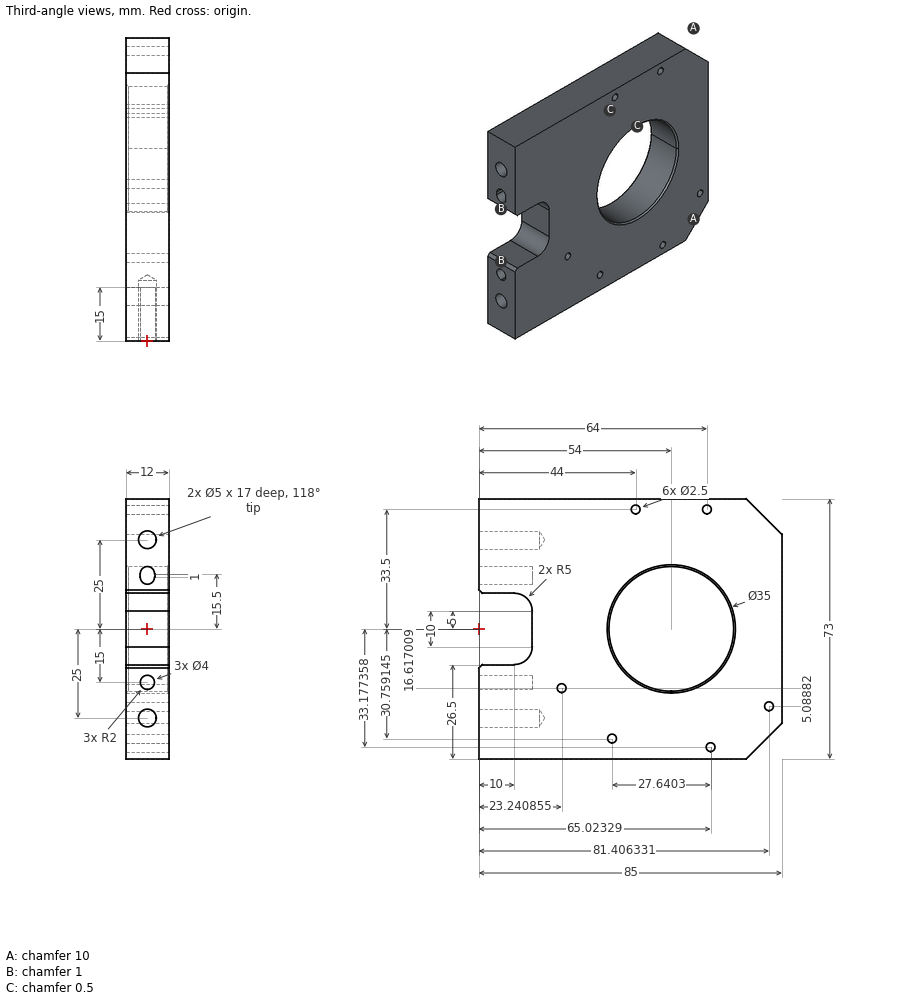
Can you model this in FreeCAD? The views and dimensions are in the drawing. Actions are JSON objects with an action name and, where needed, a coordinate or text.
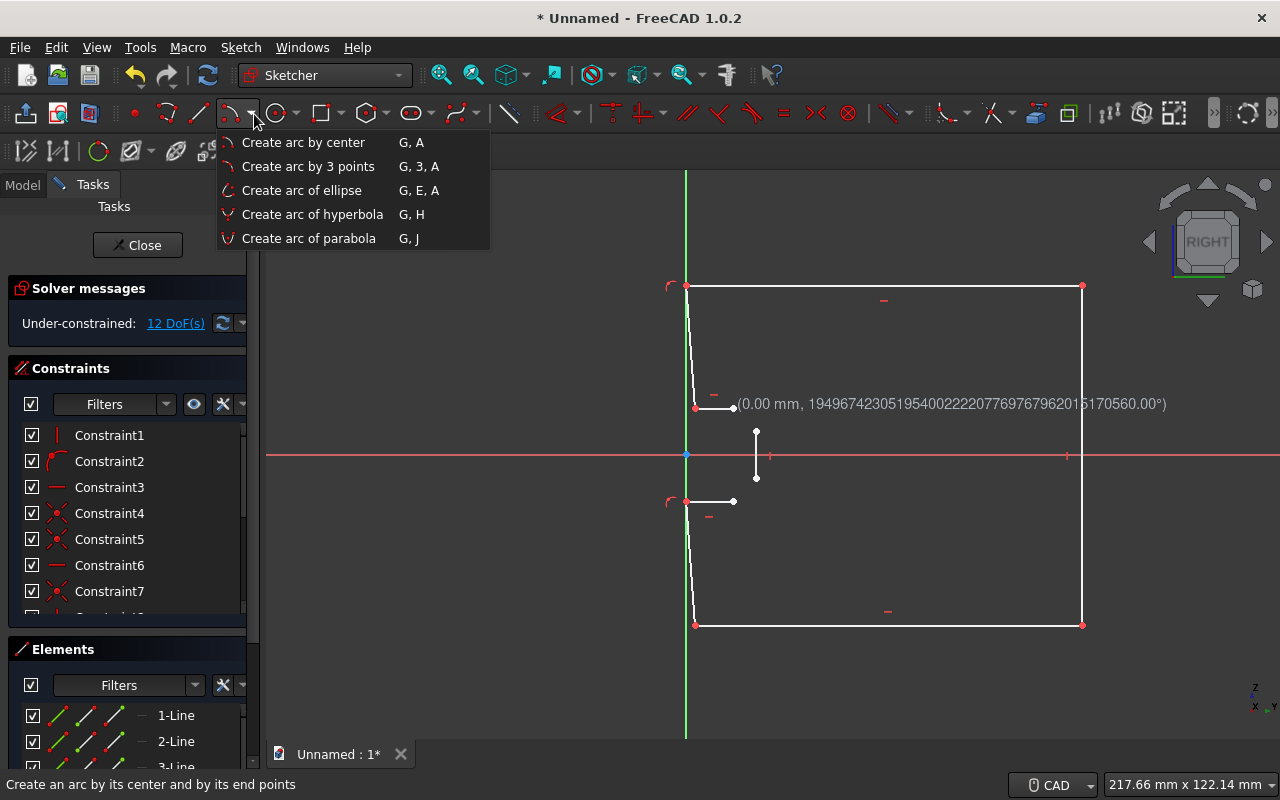
{"action": "left_click", "coordinate": [354, 166]}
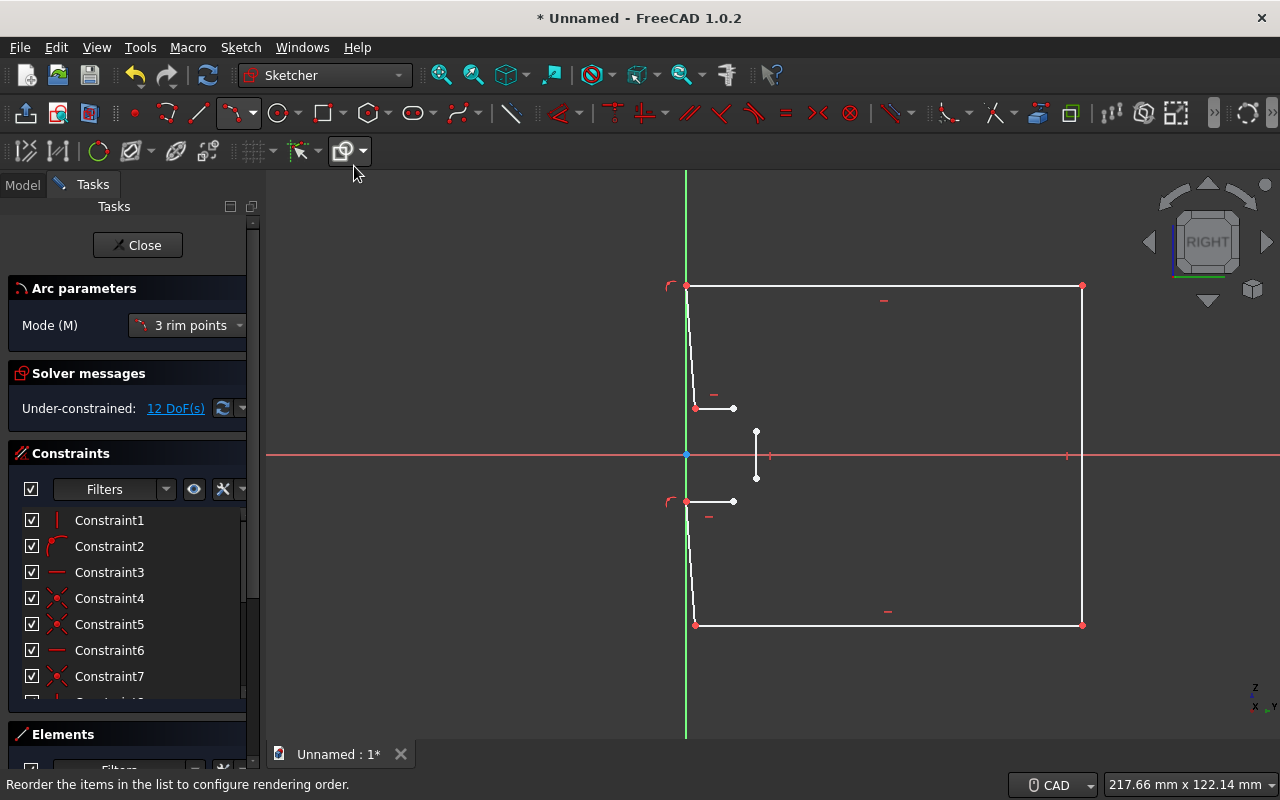
{"action": "left_click", "coordinate": [756, 479]}
{"action": "left_click", "coordinate": [733, 502]}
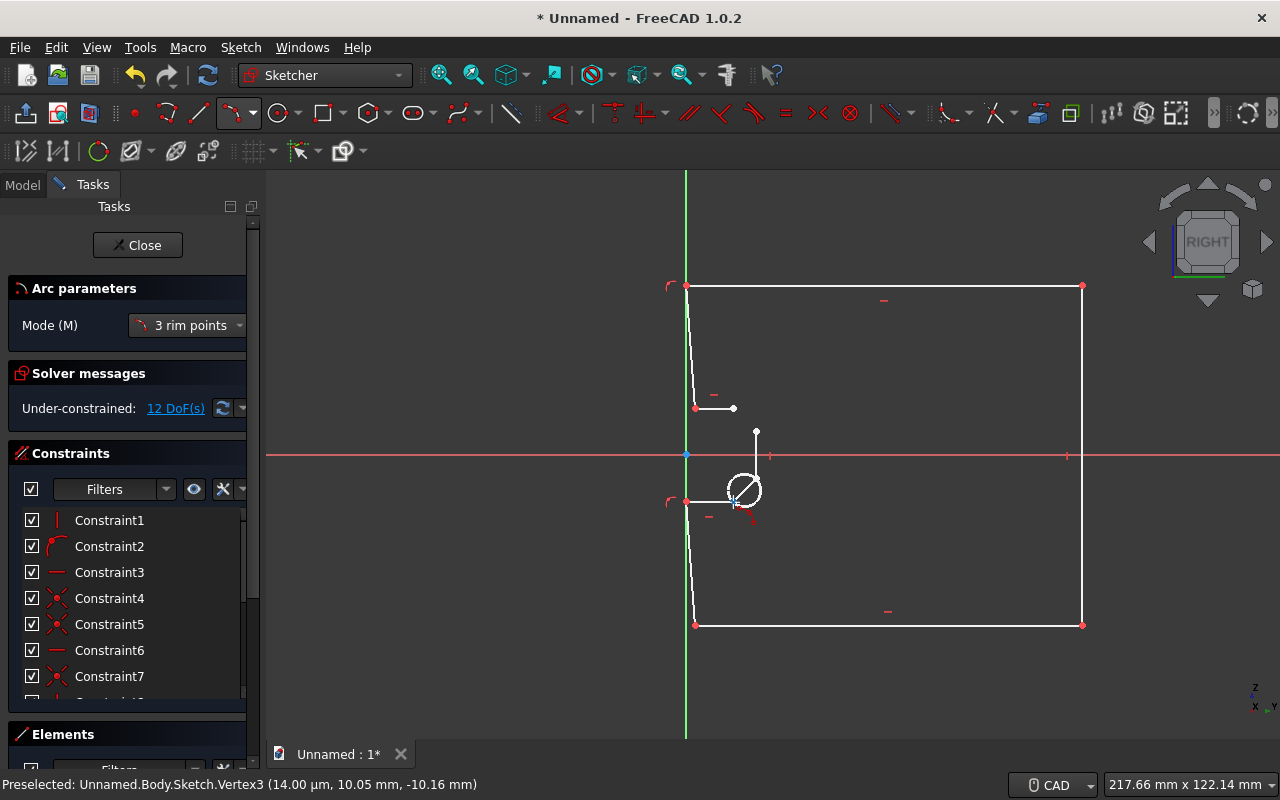
{"action": "scroll", "coordinate": [749, 494], "scroll_direction": "up", "scroll_amount": 5}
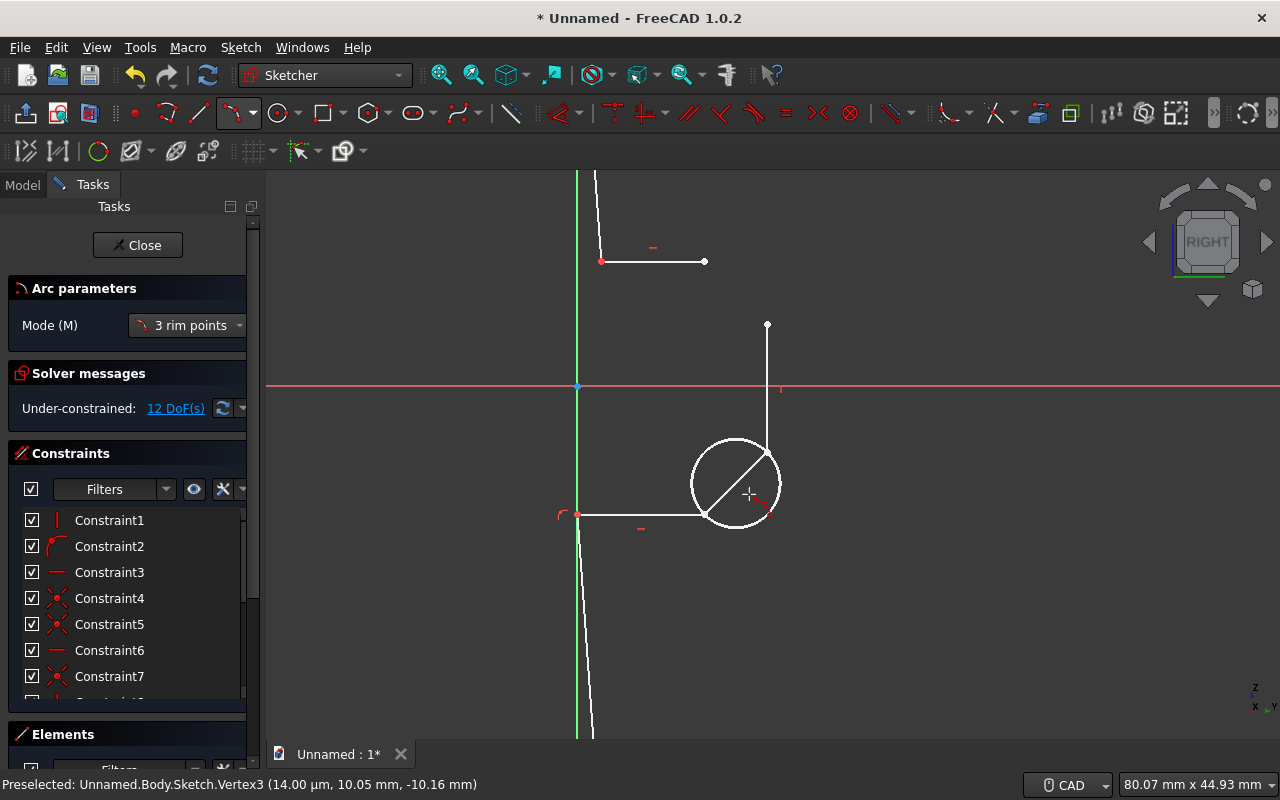
{"action": "left_click", "coordinate": [749, 494]}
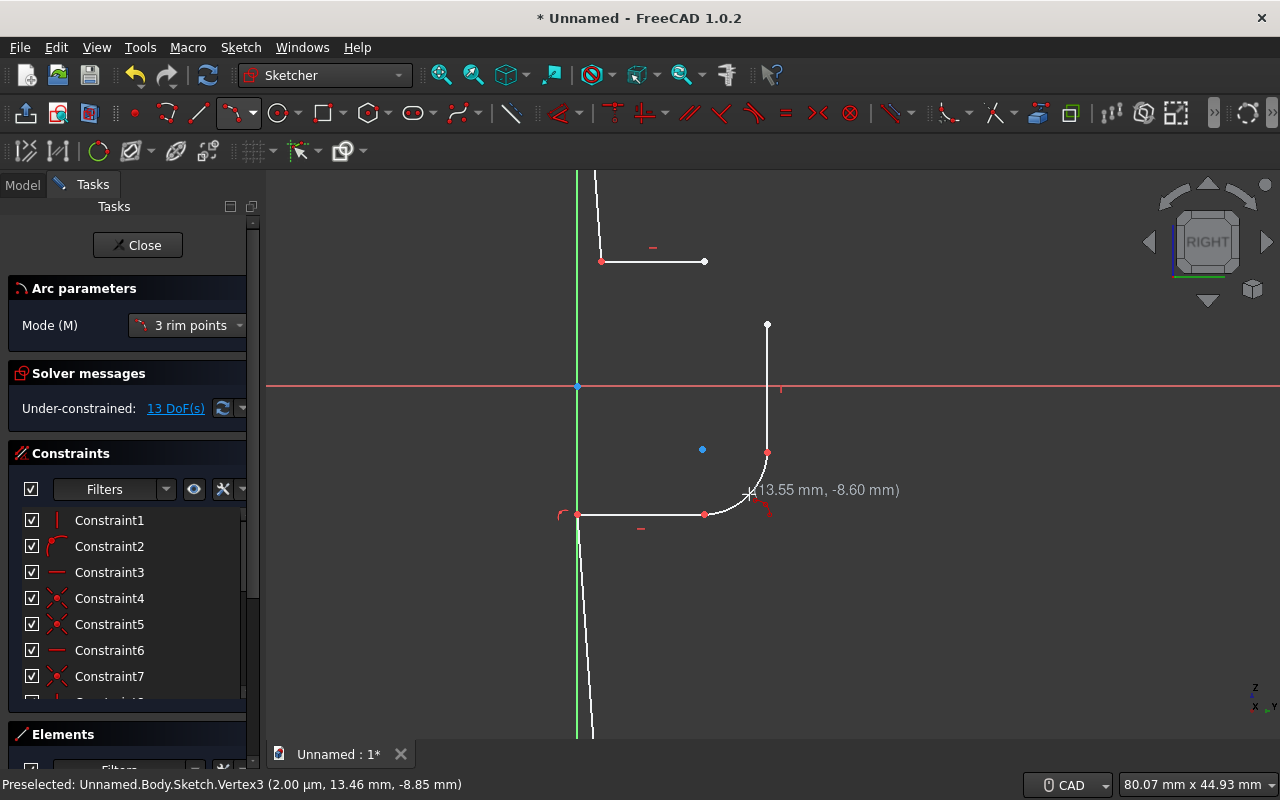
{"action": "left_click", "coordinate": [705, 262]}
{"action": "left_click", "coordinate": [767, 324]}
{"action": "left_click", "coordinate": [749, 278]}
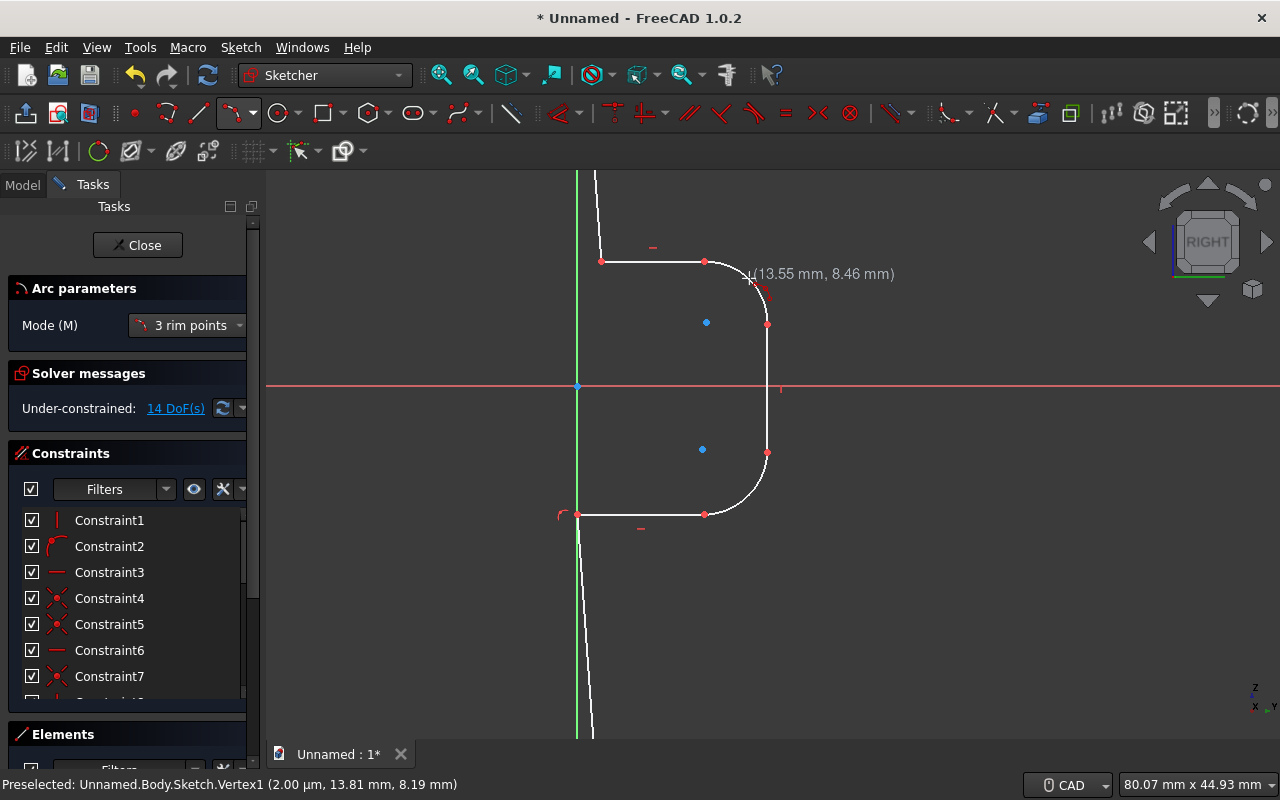
{"action": "left_click", "coordinate": [278, 114]}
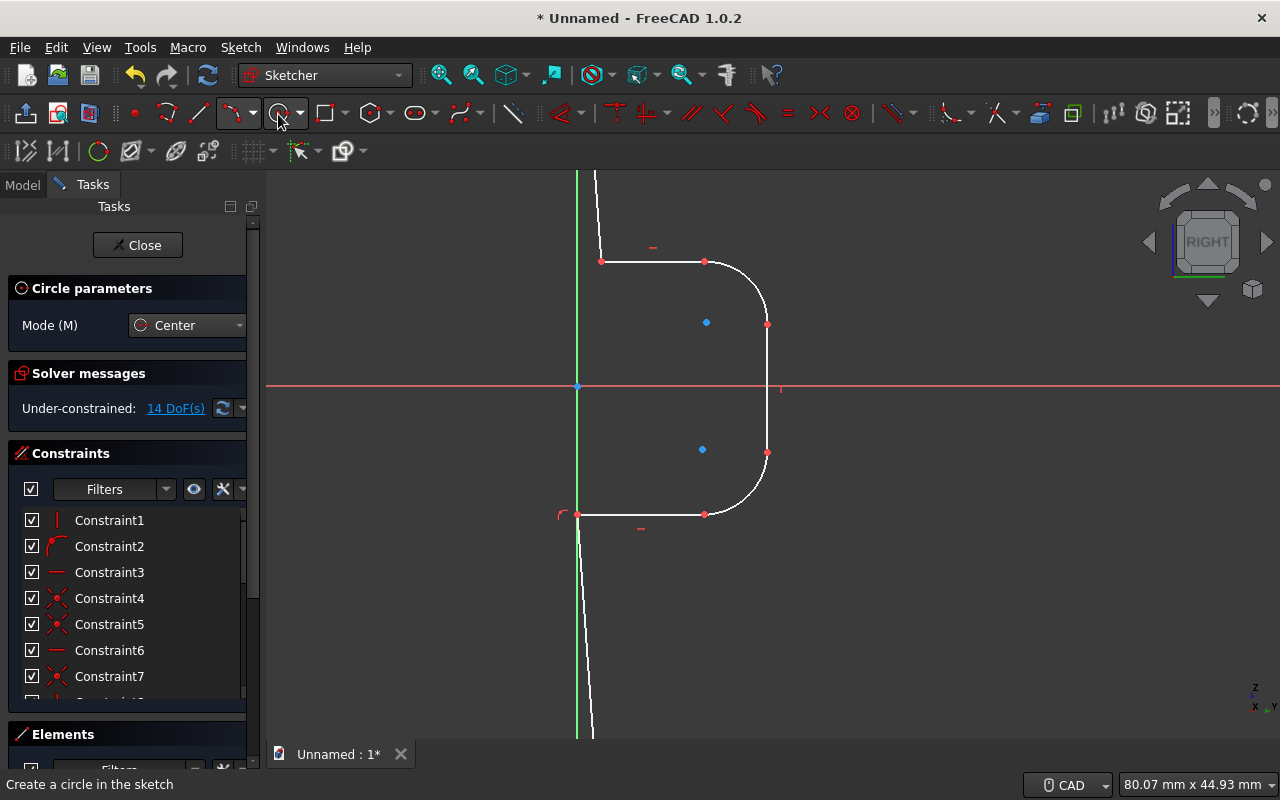
{"action": "scroll", "coordinate": [465, 494], "scroll_direction": "down", "scroll_amount": 5}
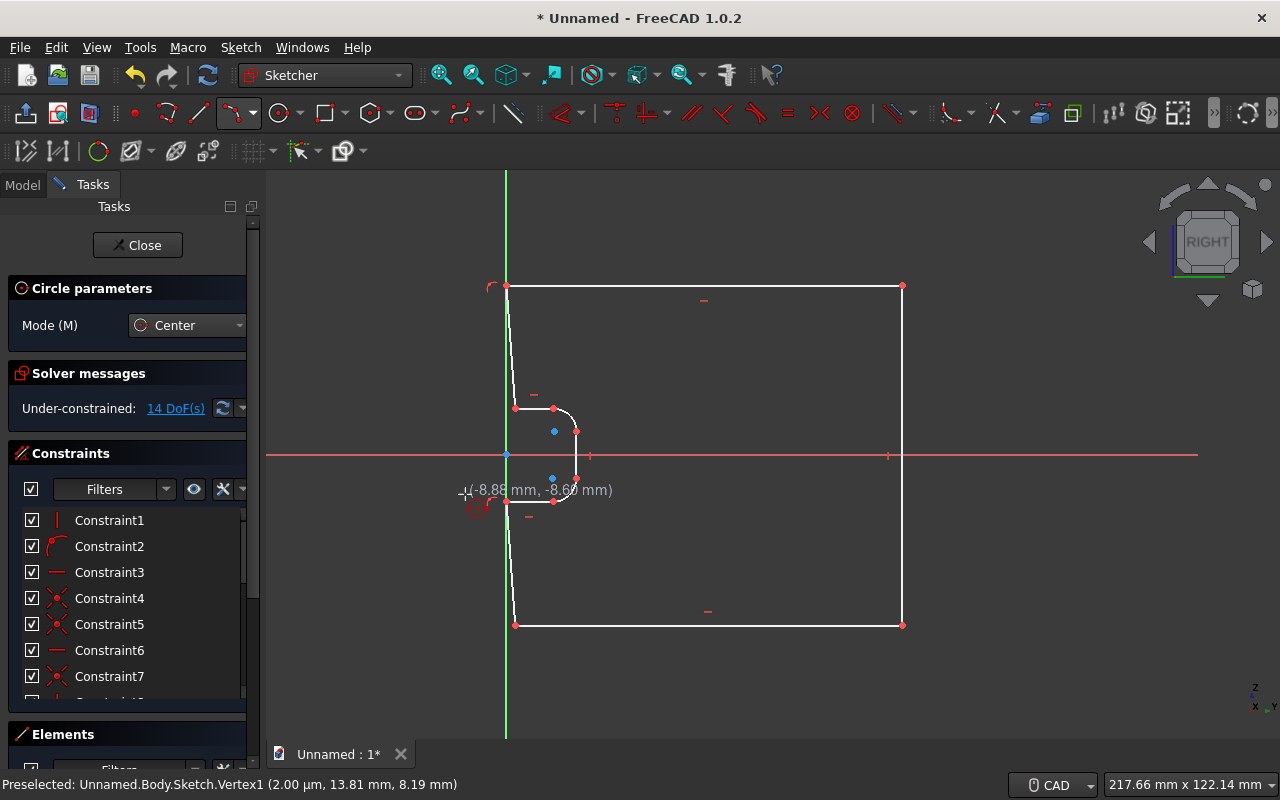
{"action": "left_click", "coordinate": [758, 455]}
{"action": "mouse_move", "coordinate": [816, 397]}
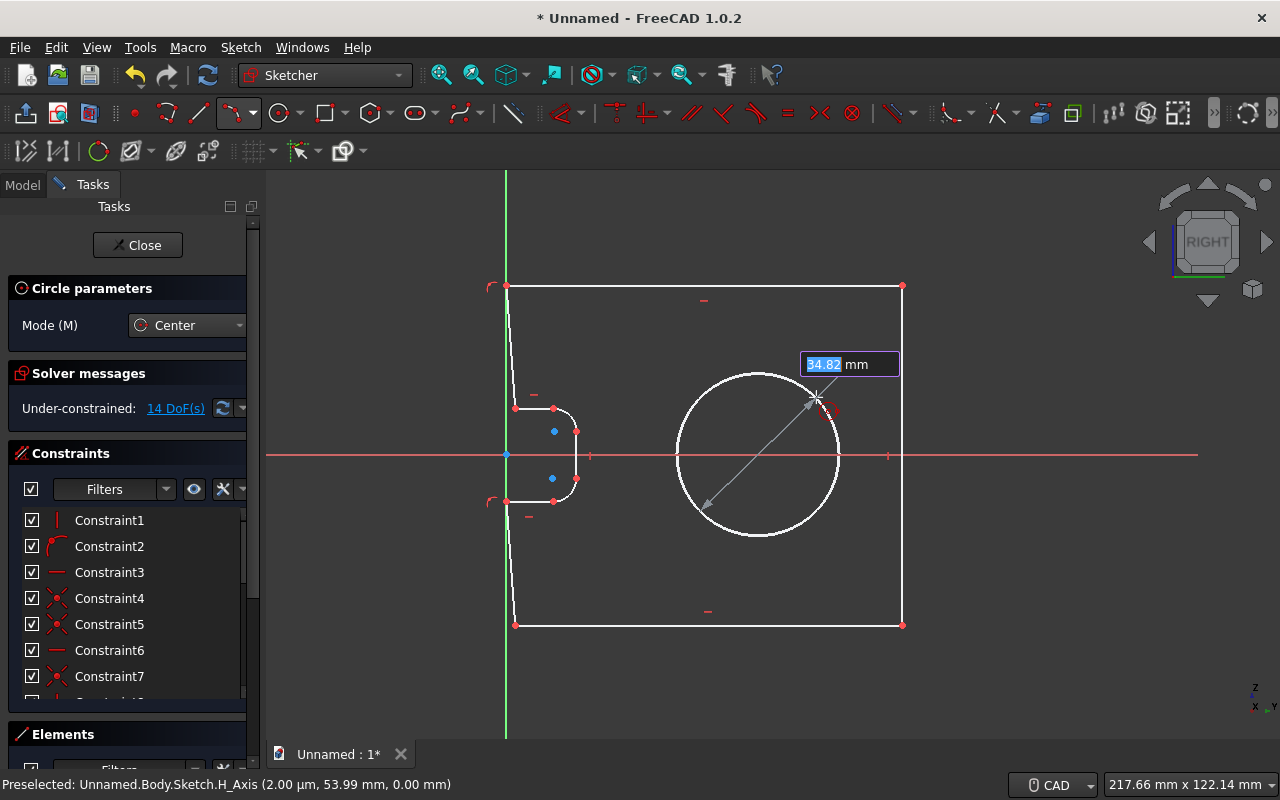
{"action": "type", "text": "35"}
{"action": "key", "text": "Return"}
{"action": "key", "text": "Escape"}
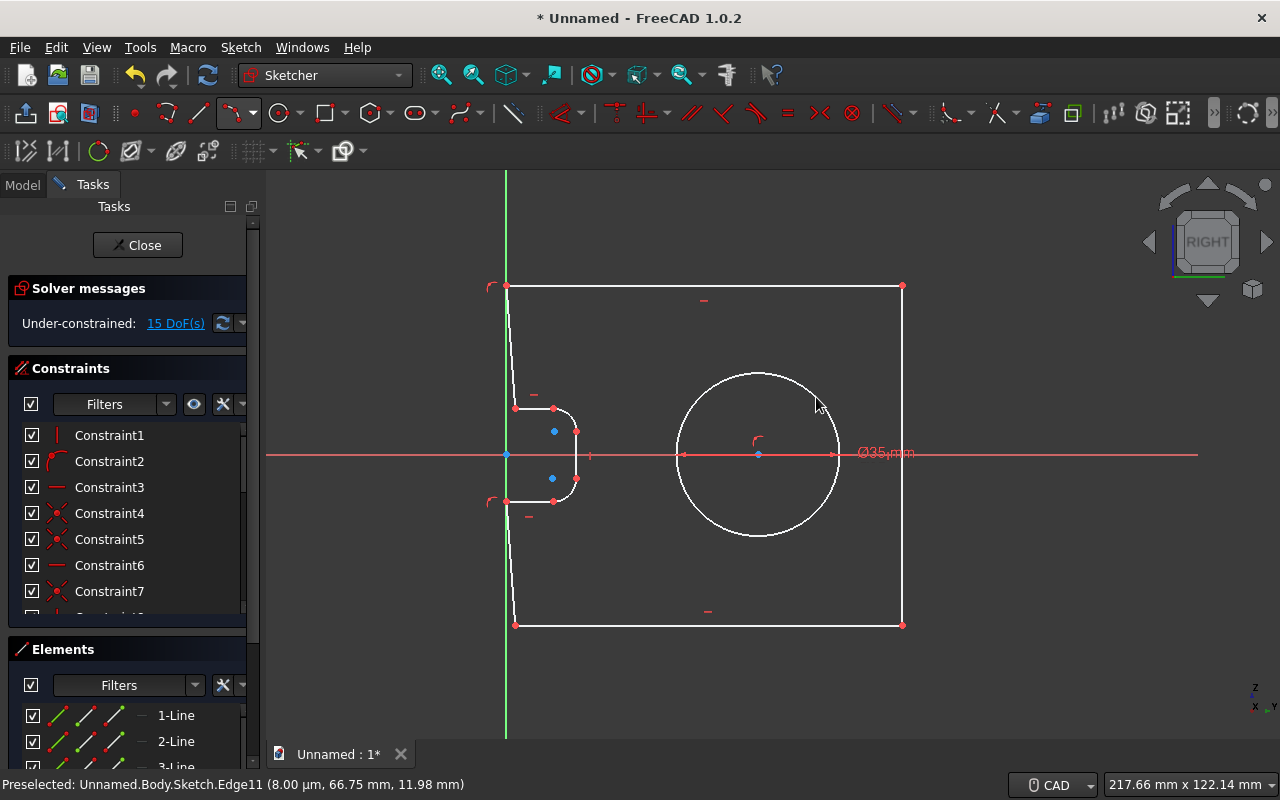
{"action": "scroll", "coordinate": [576, 465], "scroll_direction": "up", "scroll_amount": 2}